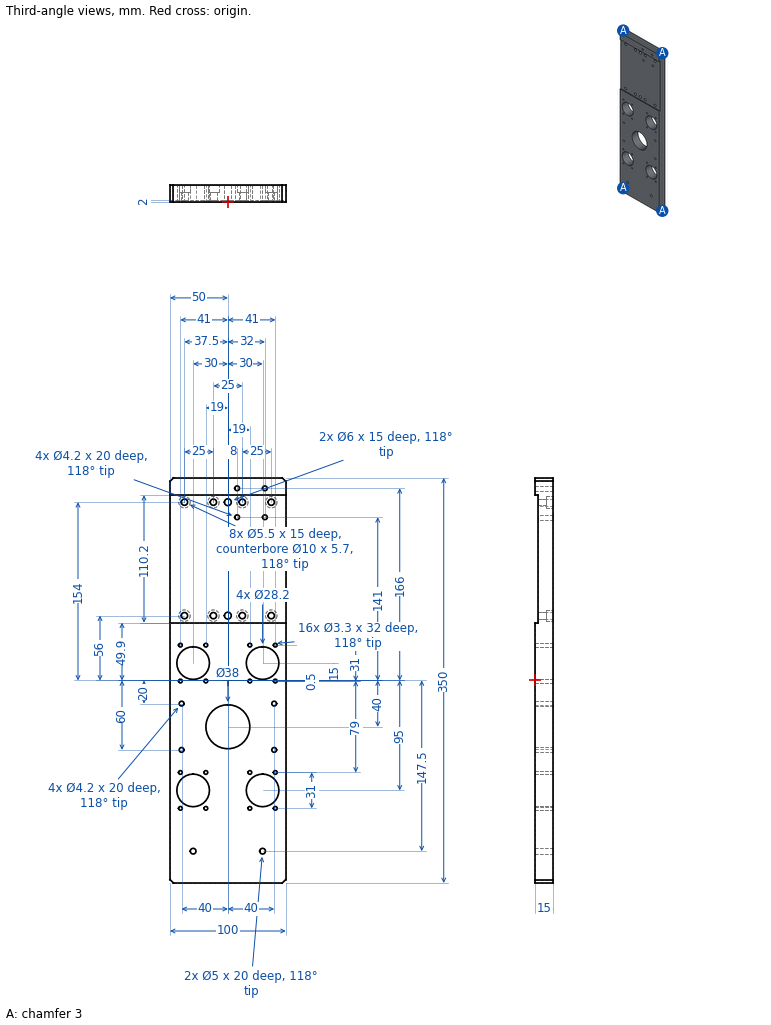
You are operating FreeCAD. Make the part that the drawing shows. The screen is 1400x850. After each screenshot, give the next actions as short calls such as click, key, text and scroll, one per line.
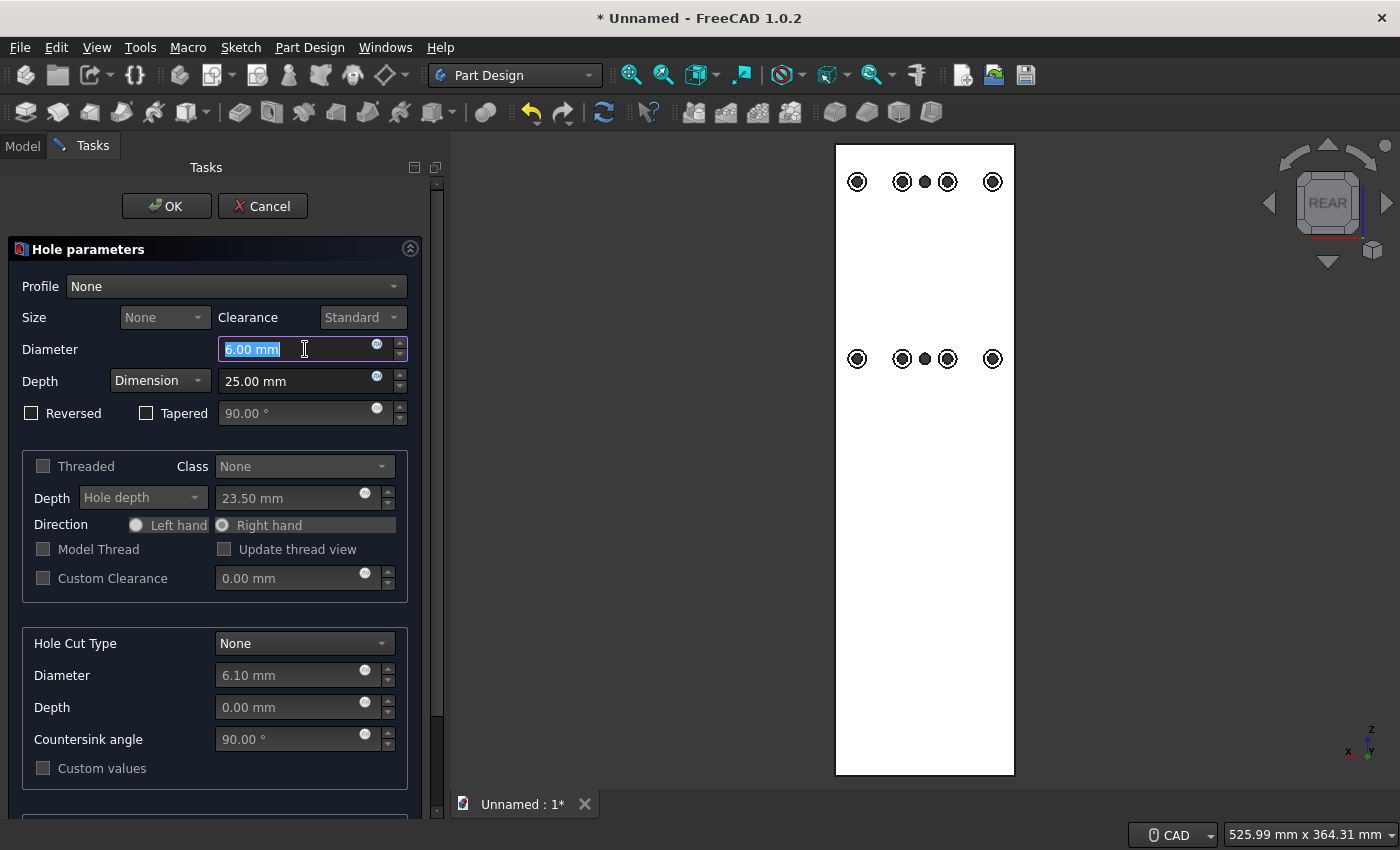
text(6)
key(Tab)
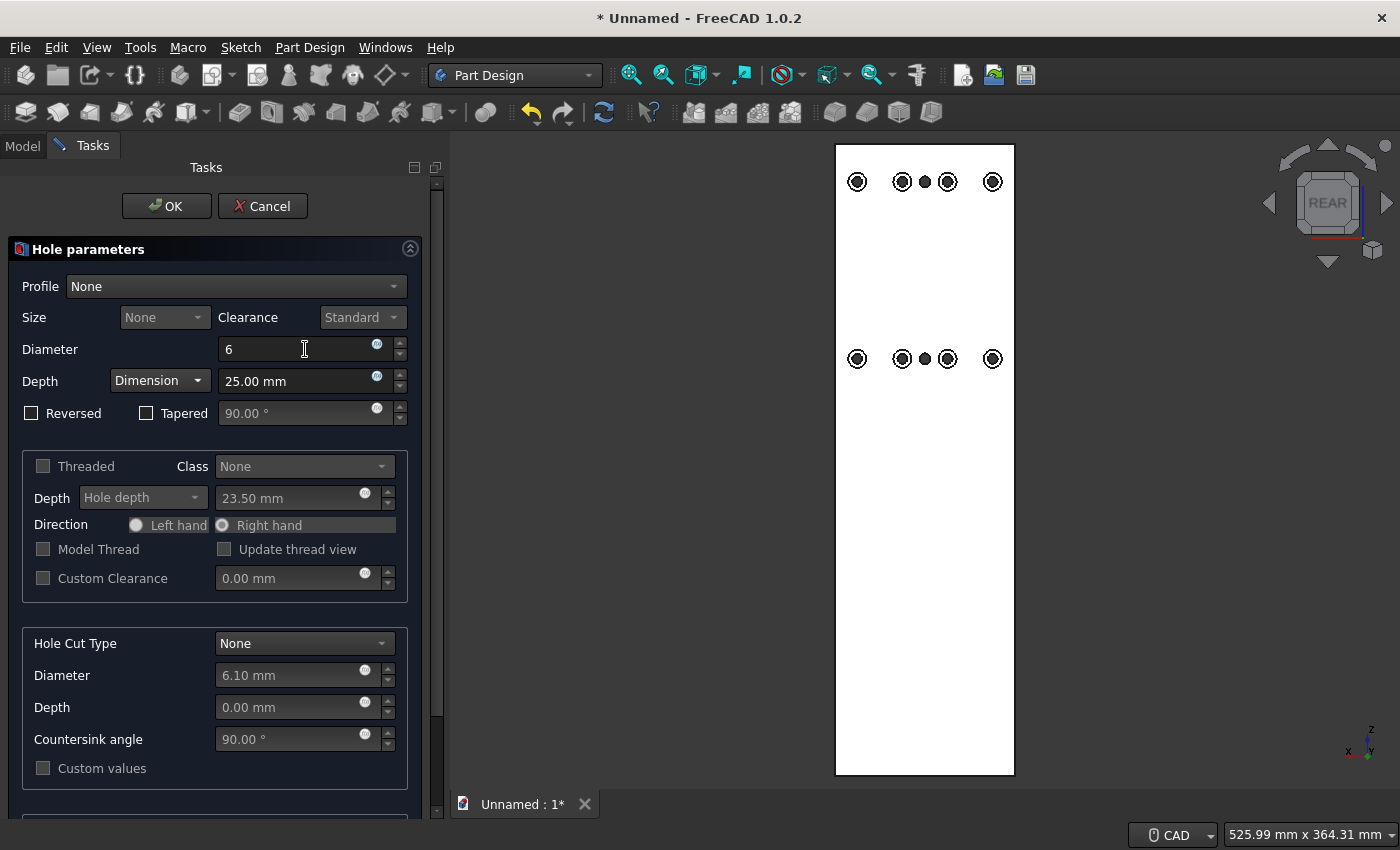
triple_click(305, 381)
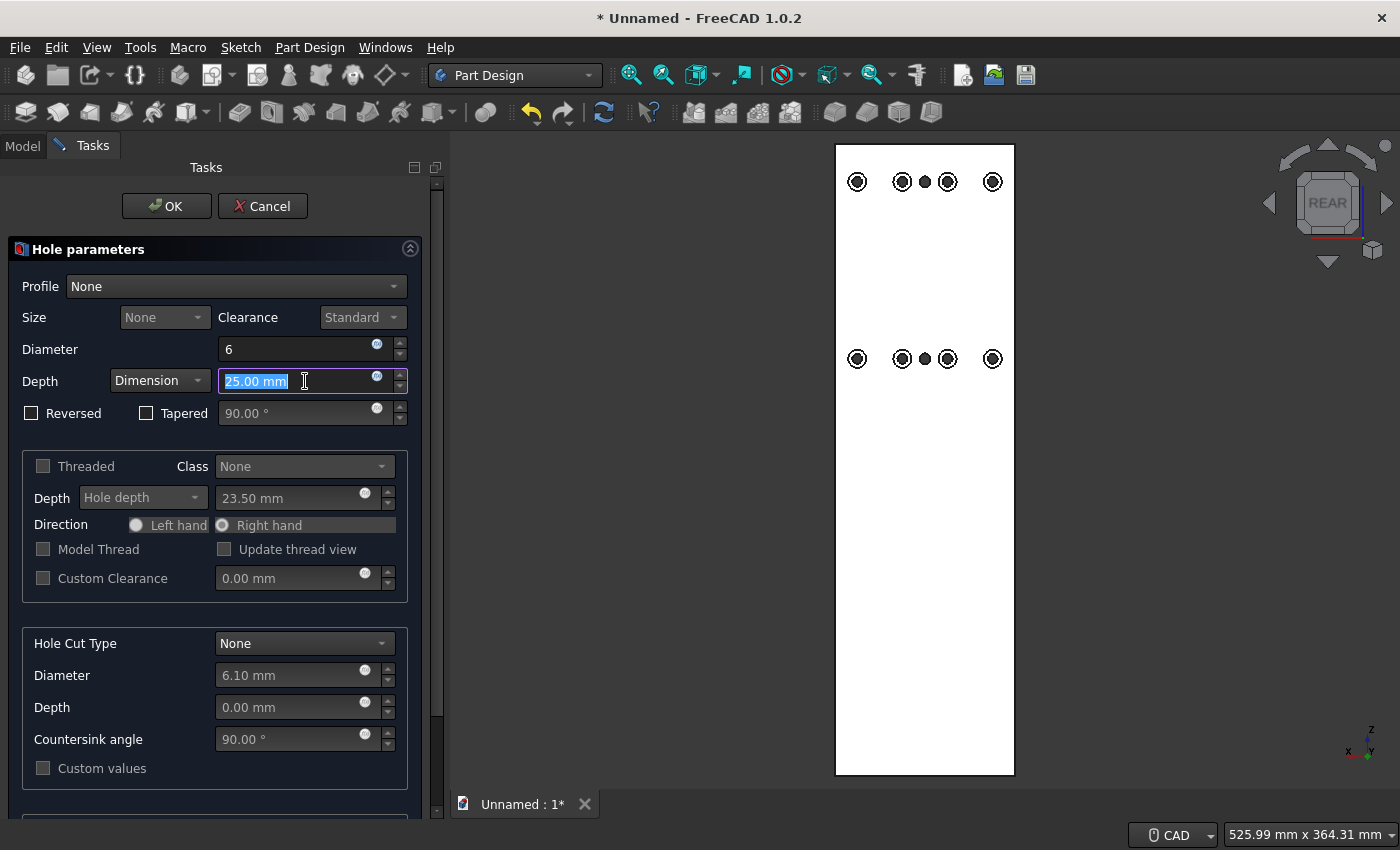
text(15)
key(Tab)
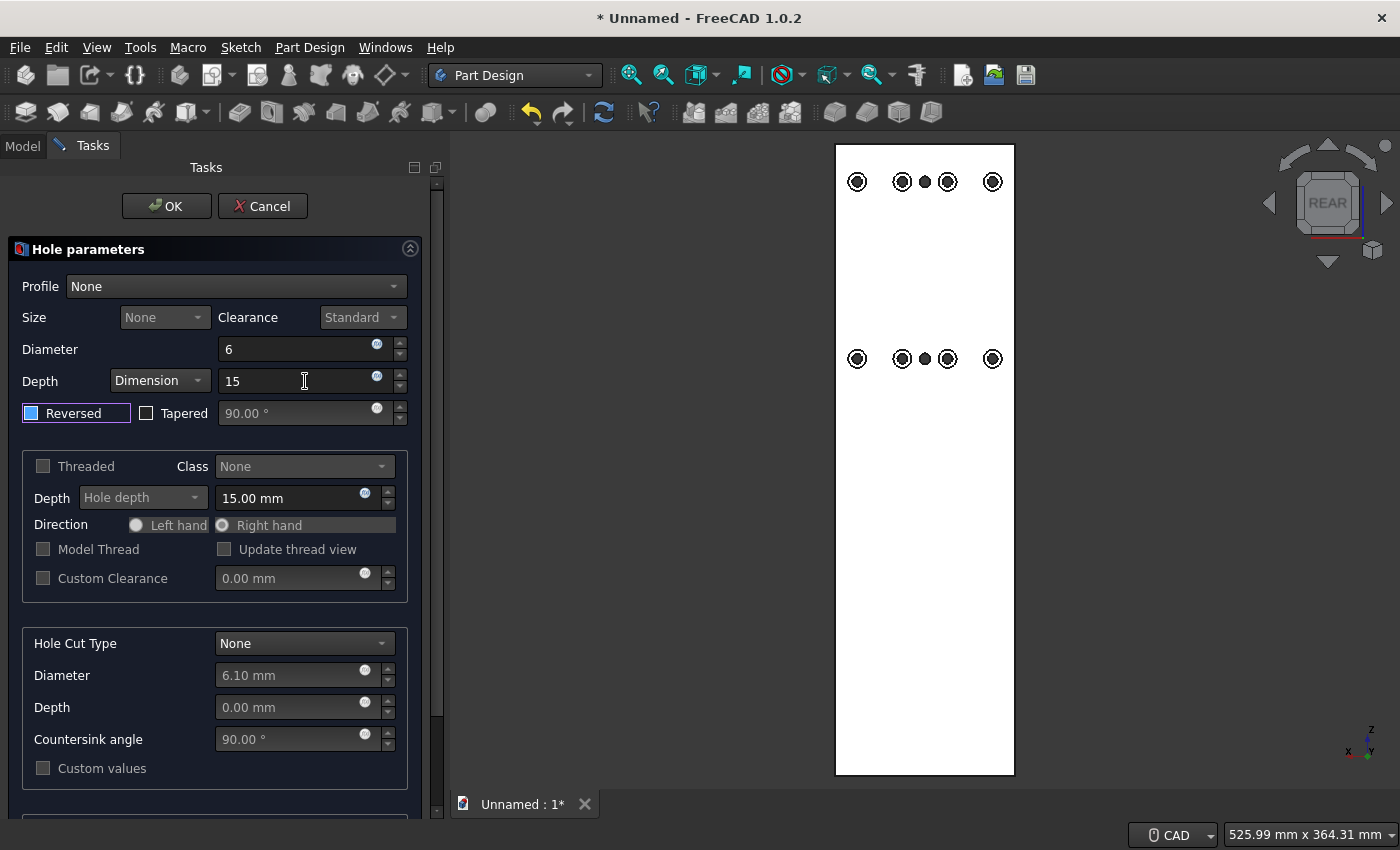
click(167, 206)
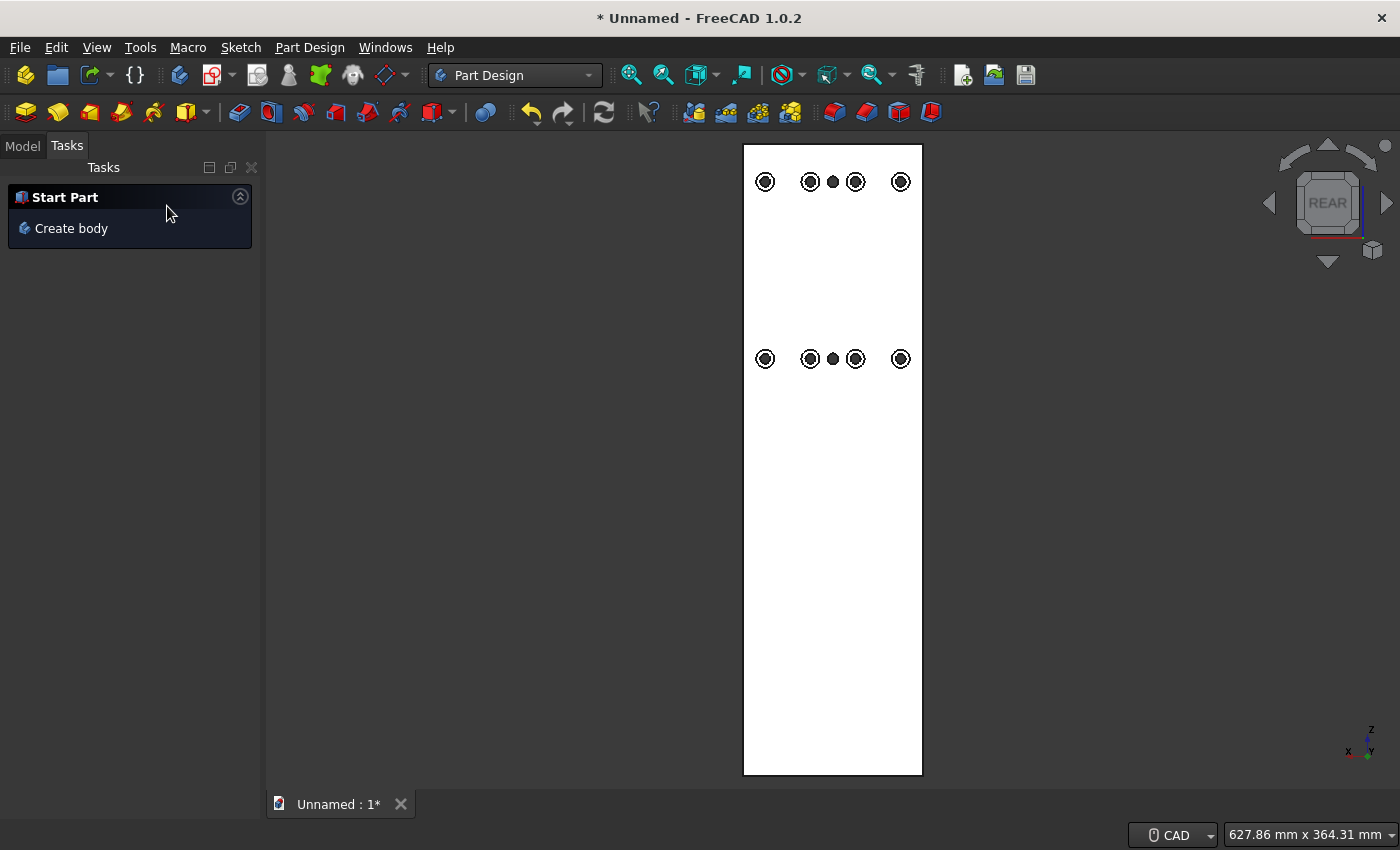
click(833, 459)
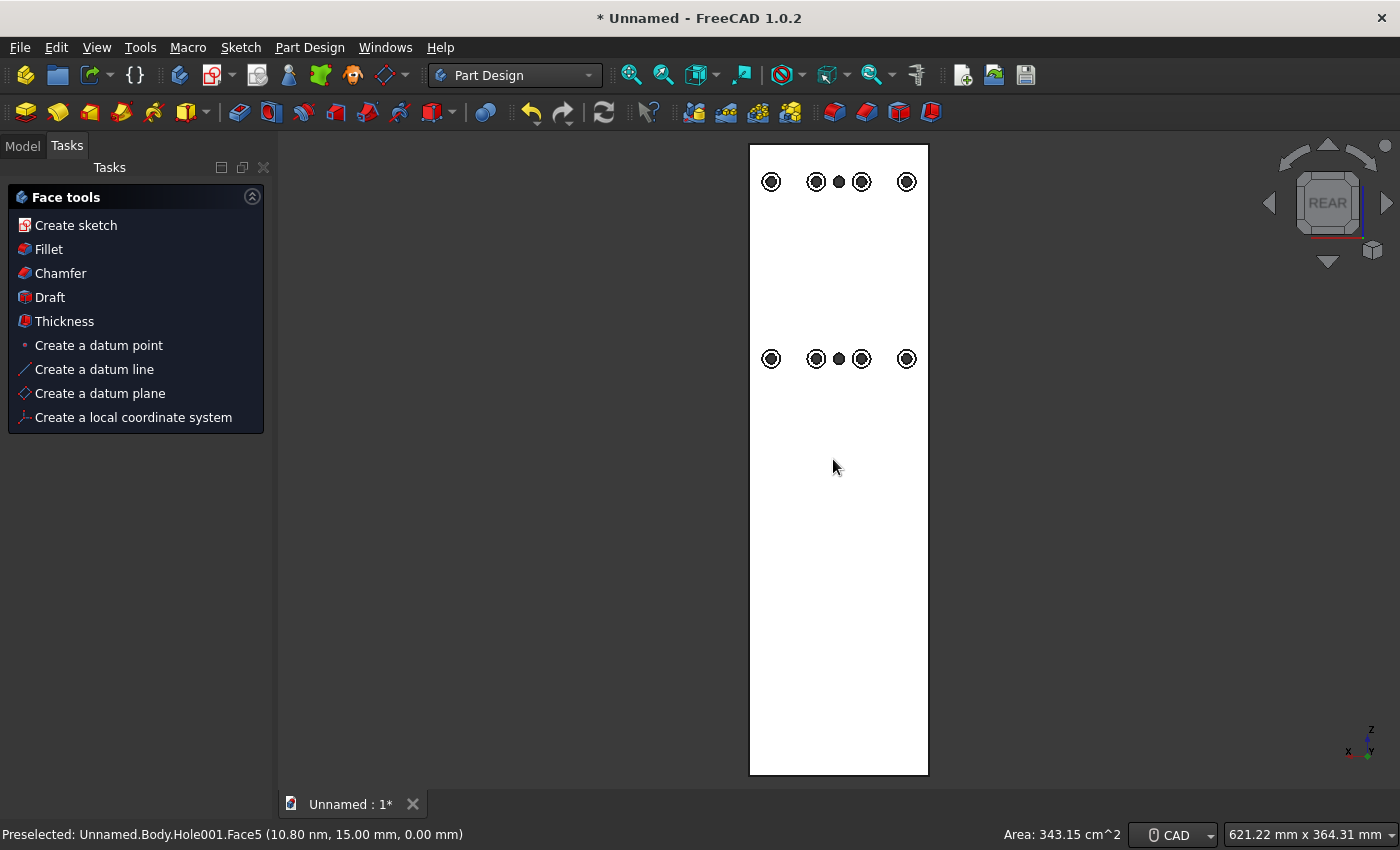
click(212, 76)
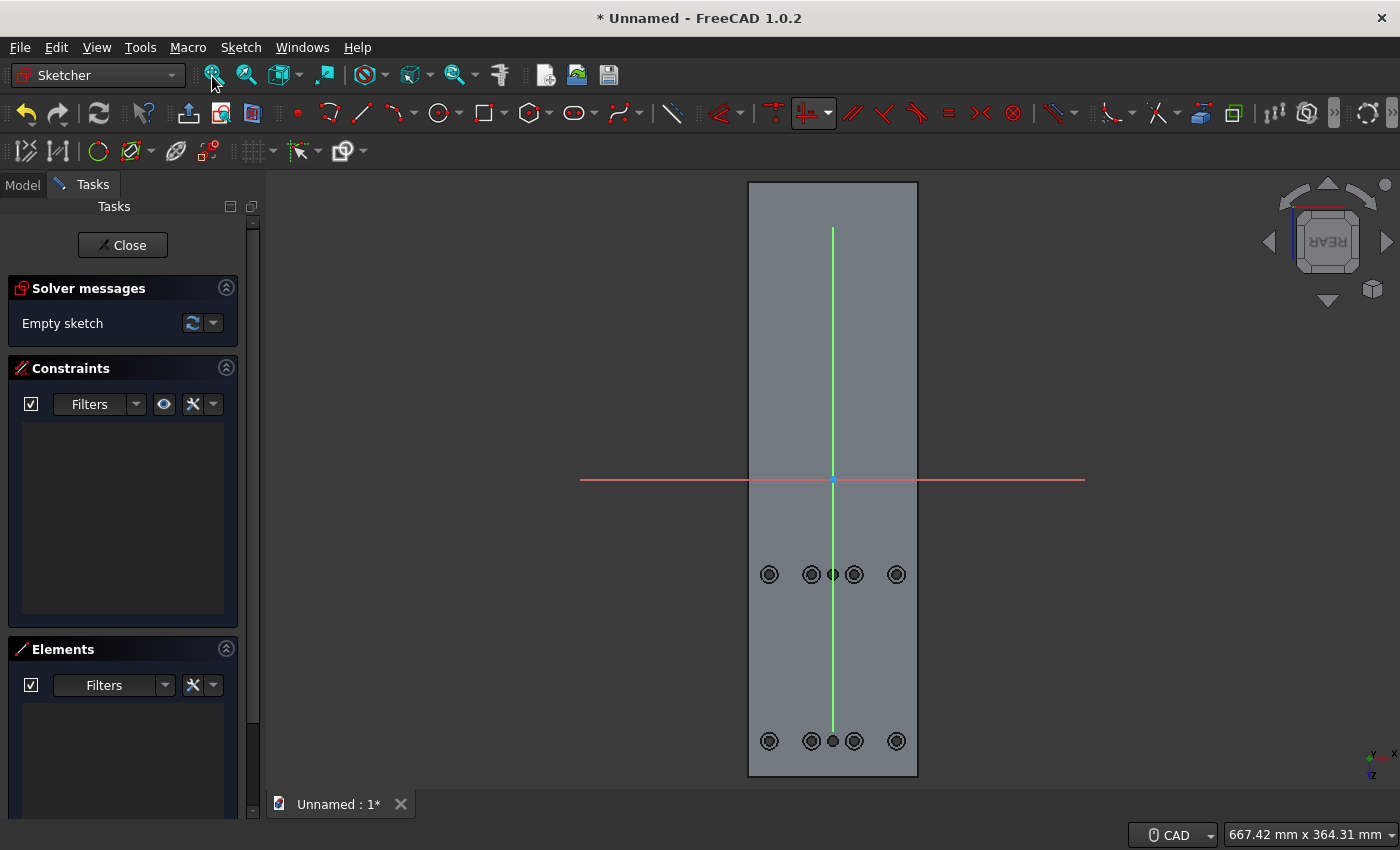
scroll(855, 413, up, 7)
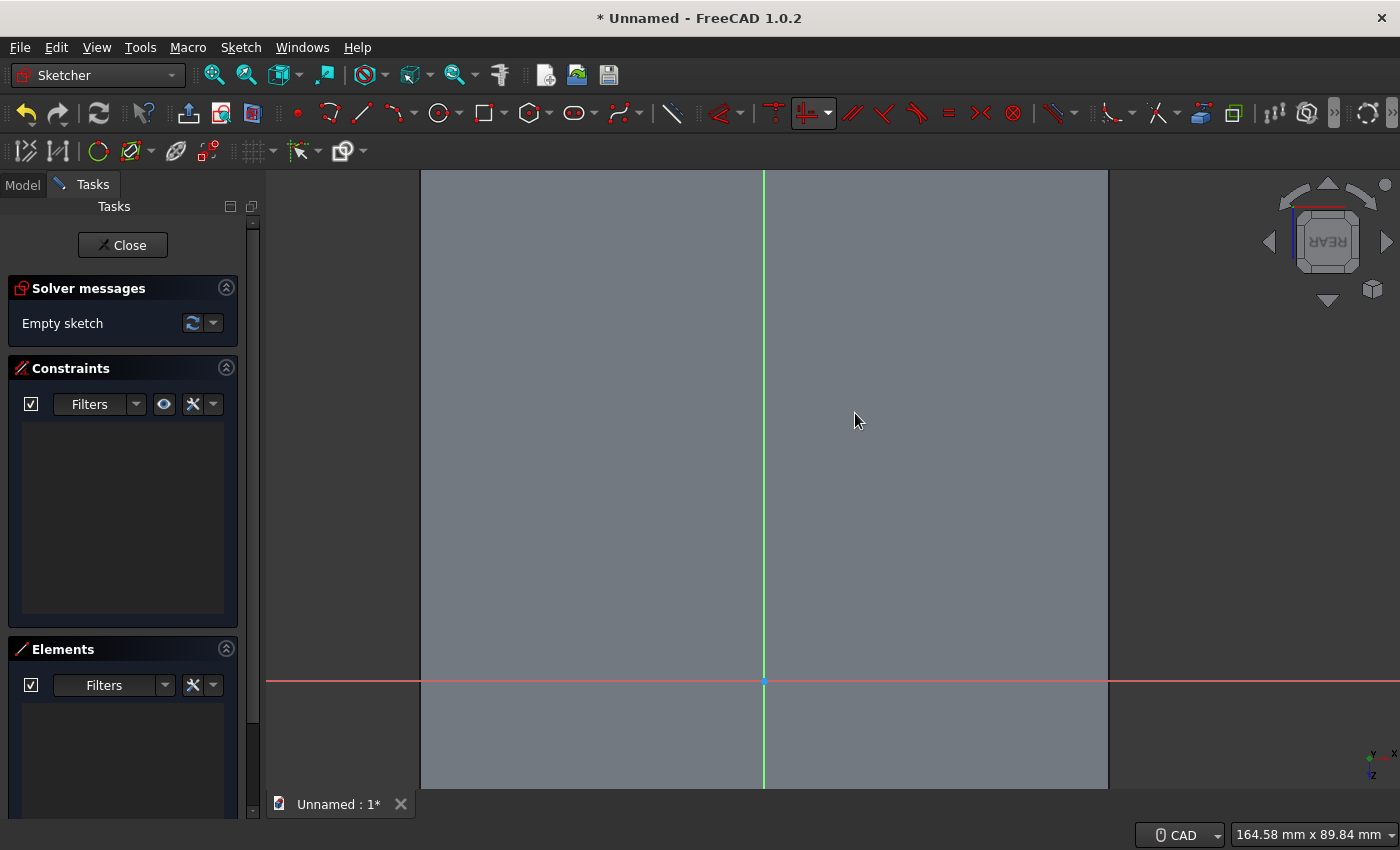
click(440, 114)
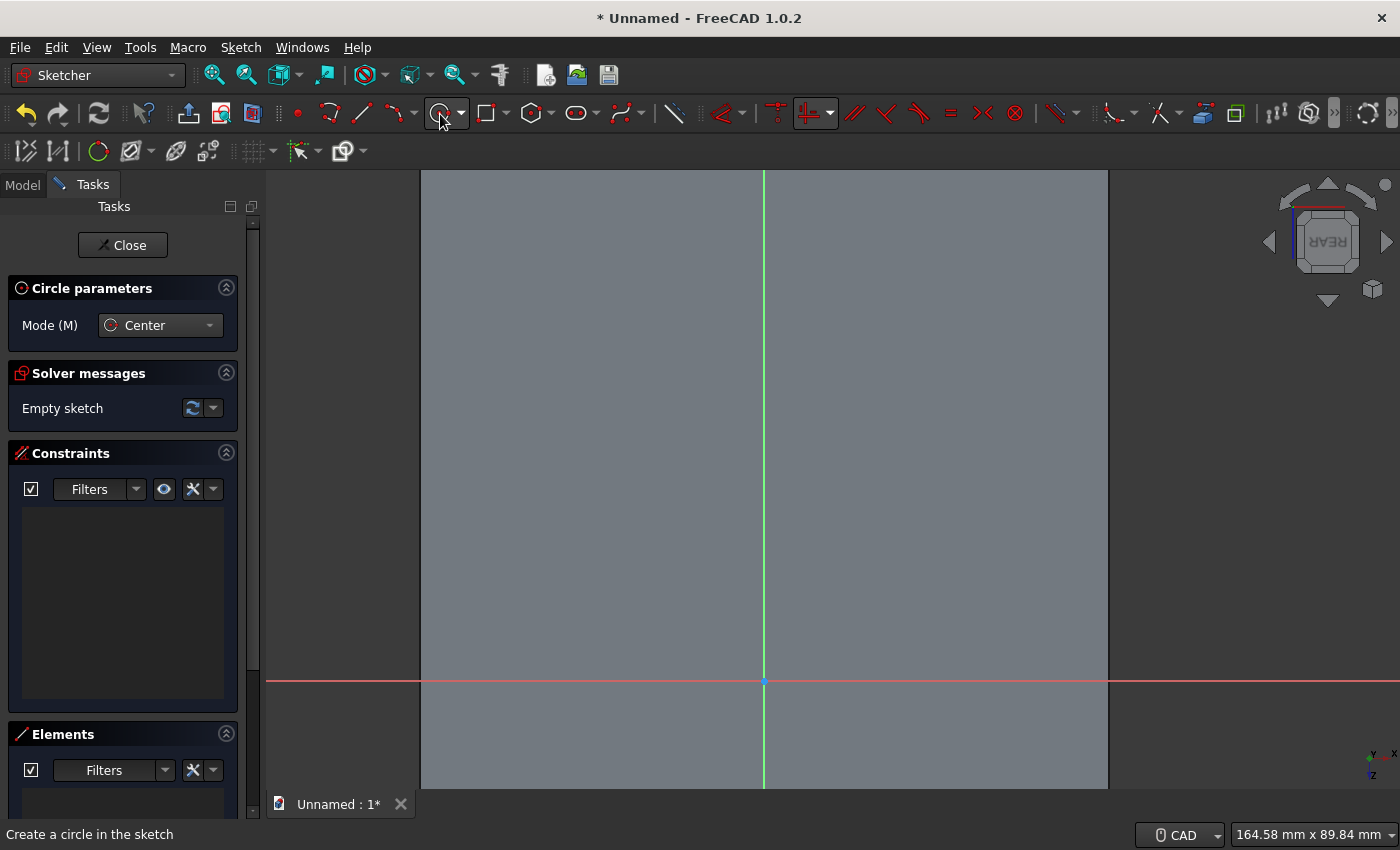
click(764, 406)
click(857, 313)
key(Escape)